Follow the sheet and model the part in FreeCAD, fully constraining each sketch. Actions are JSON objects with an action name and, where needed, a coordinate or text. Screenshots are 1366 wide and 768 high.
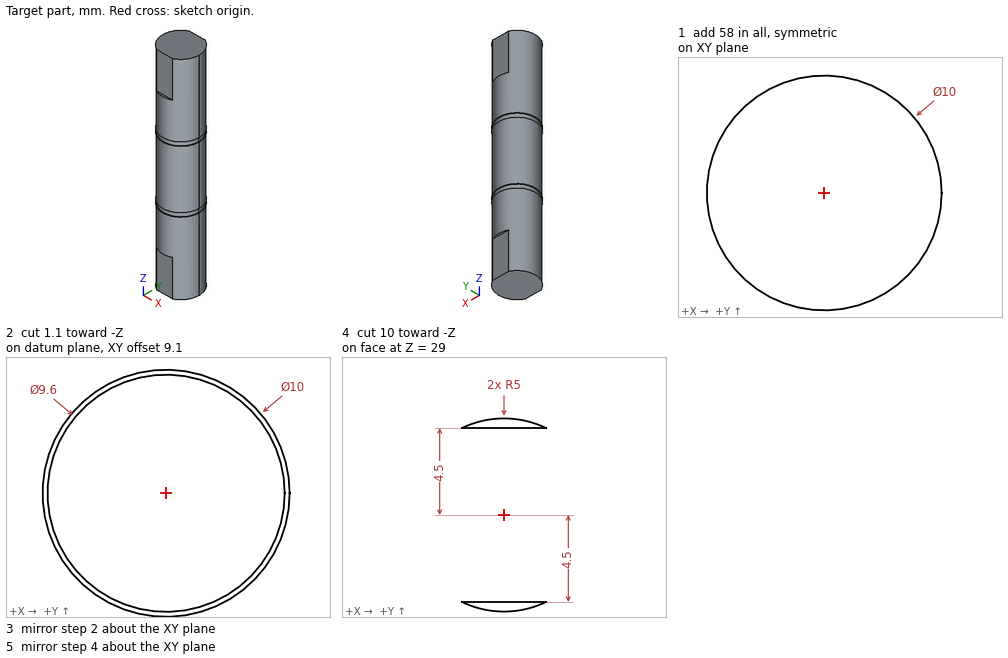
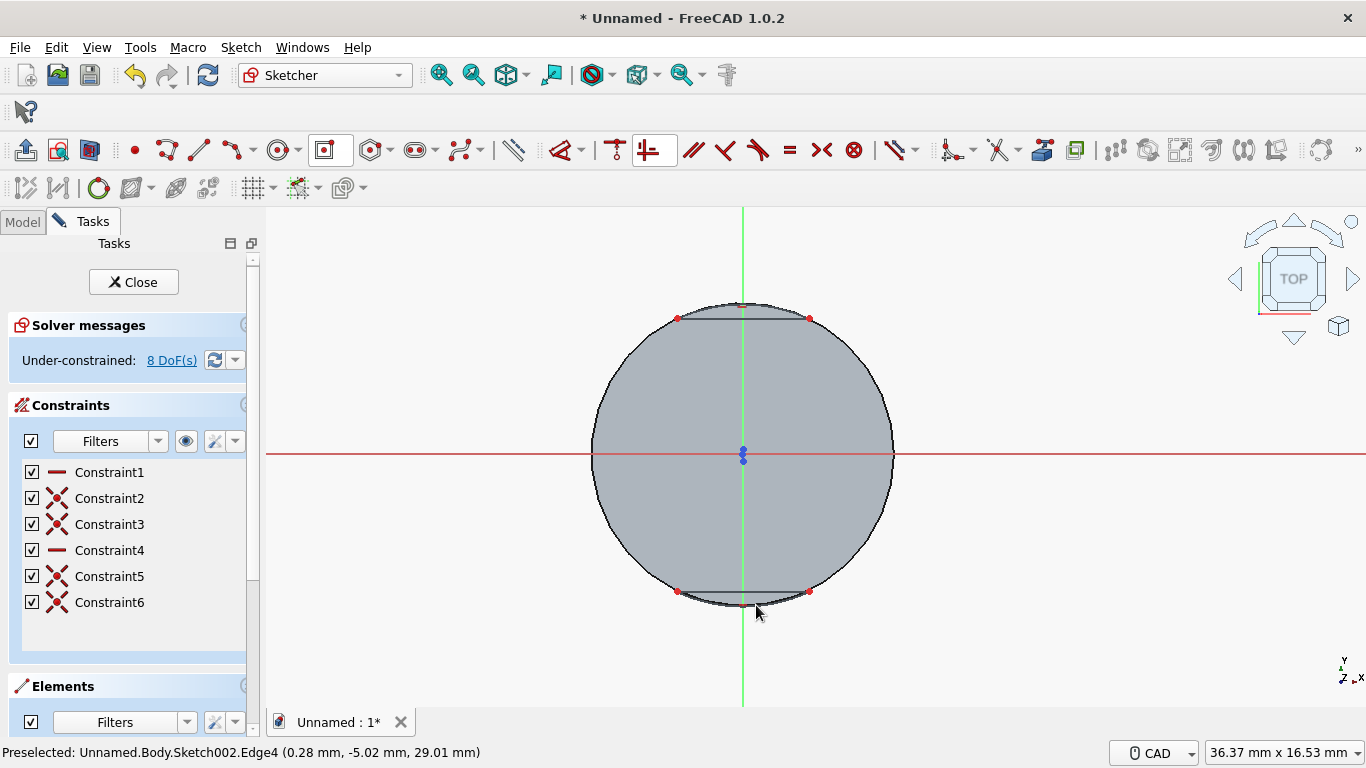
{"action": "left_click", "coordinate": [770, 307]}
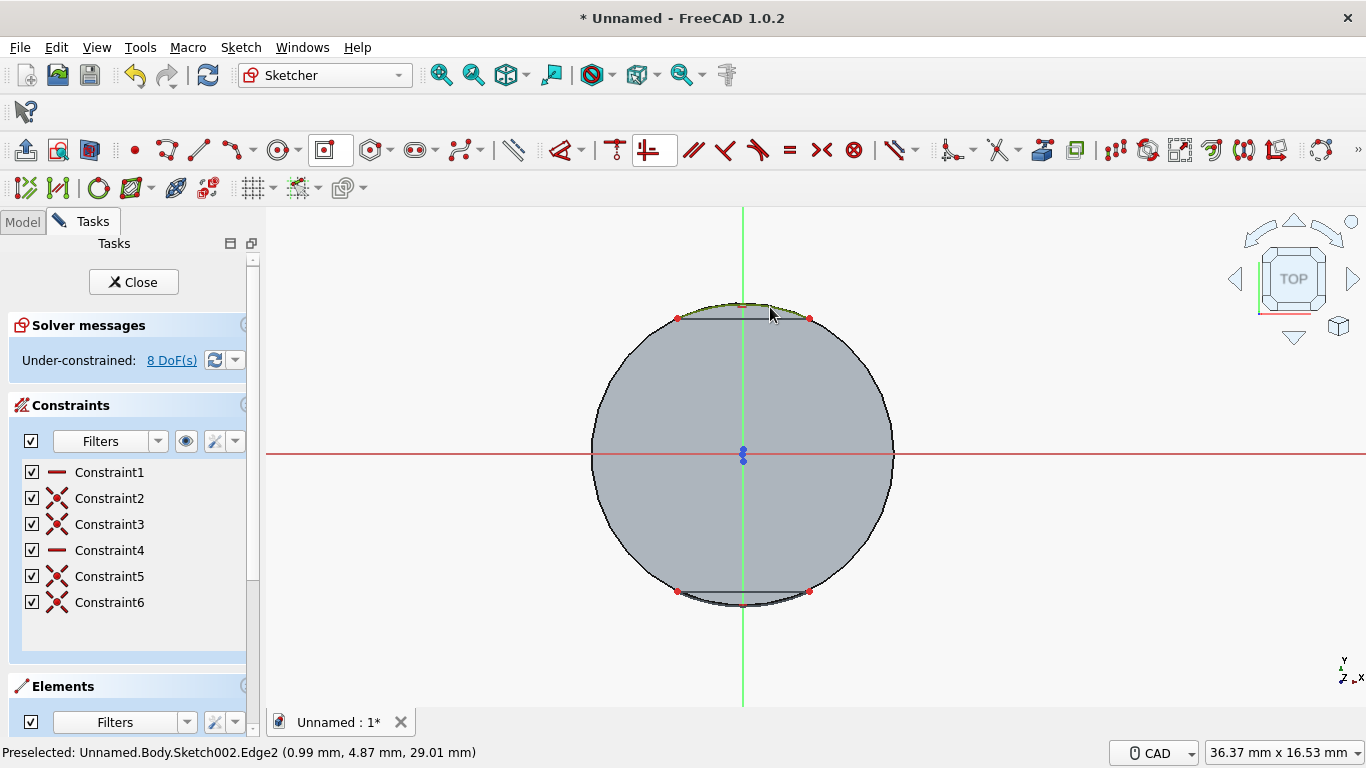
{"action": "left_click", "coordinate": [716, 604]}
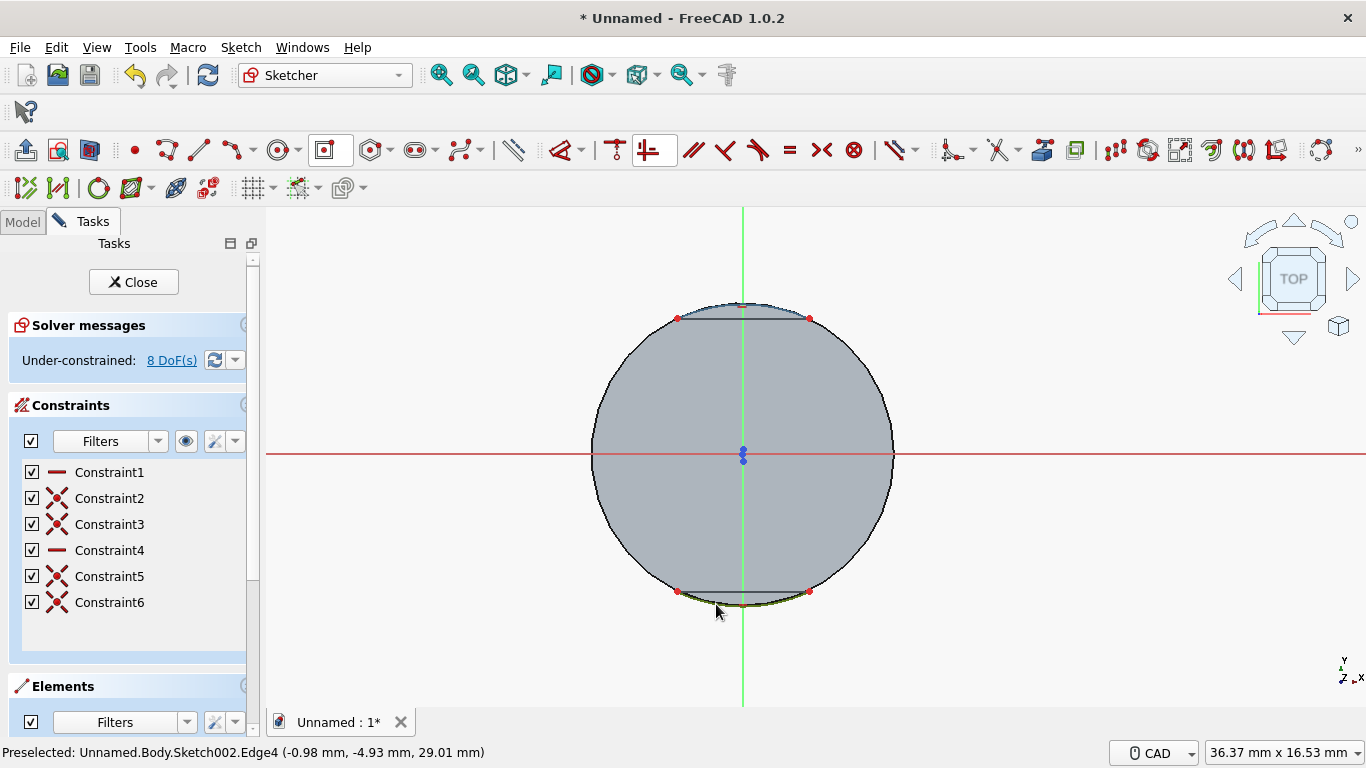
{"action": "left_click", "coordinate": [616, 150]}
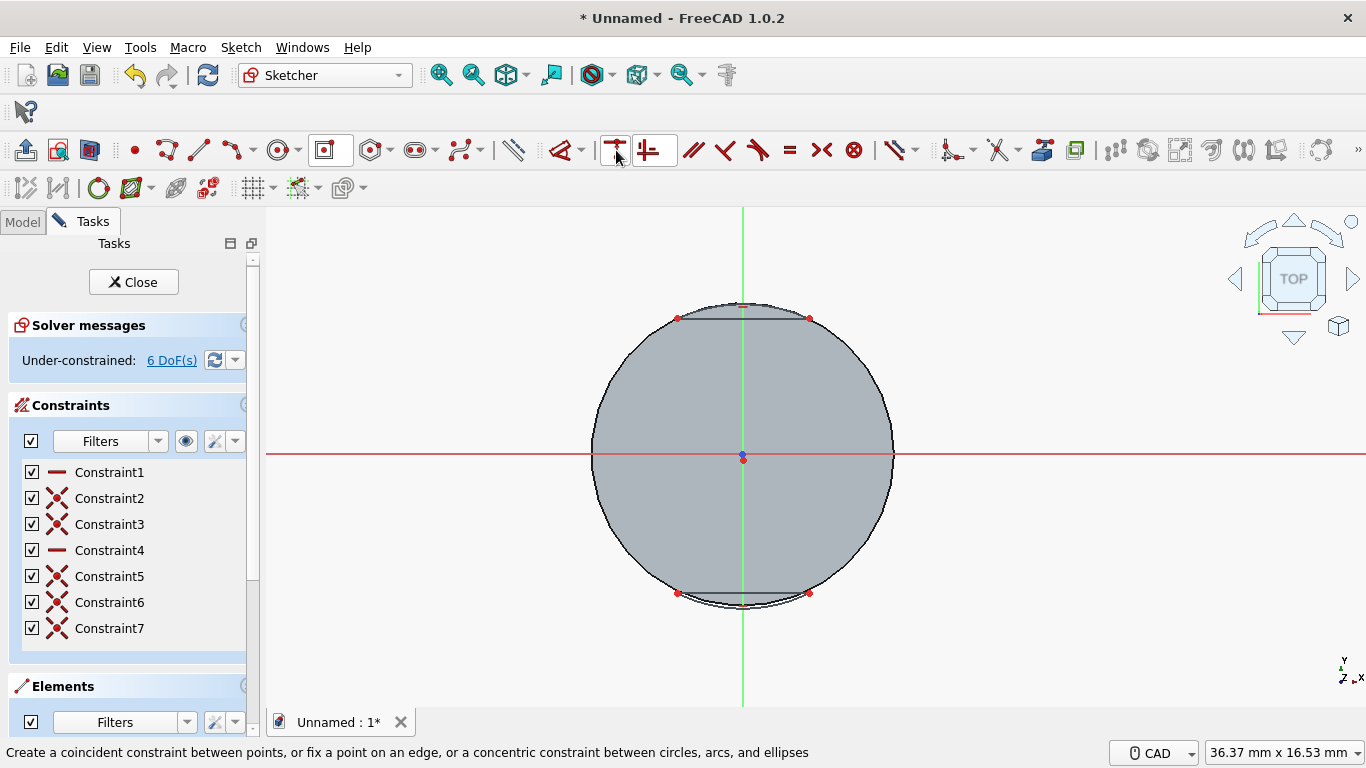
{"action": "left_click_drag", "start_coordinate": [733, 444], "coordinate": [753, 470]}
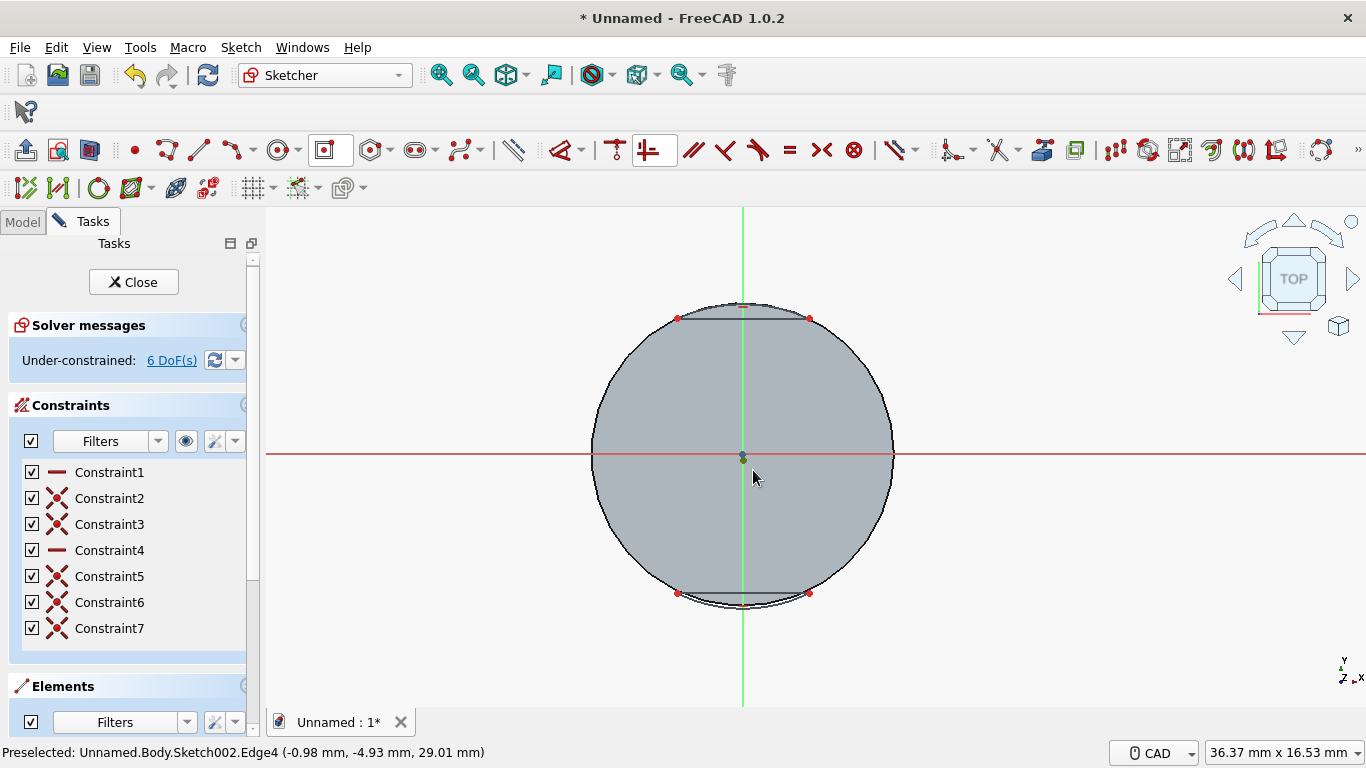
{"action": "left_click", "coordinate": [616, 150]}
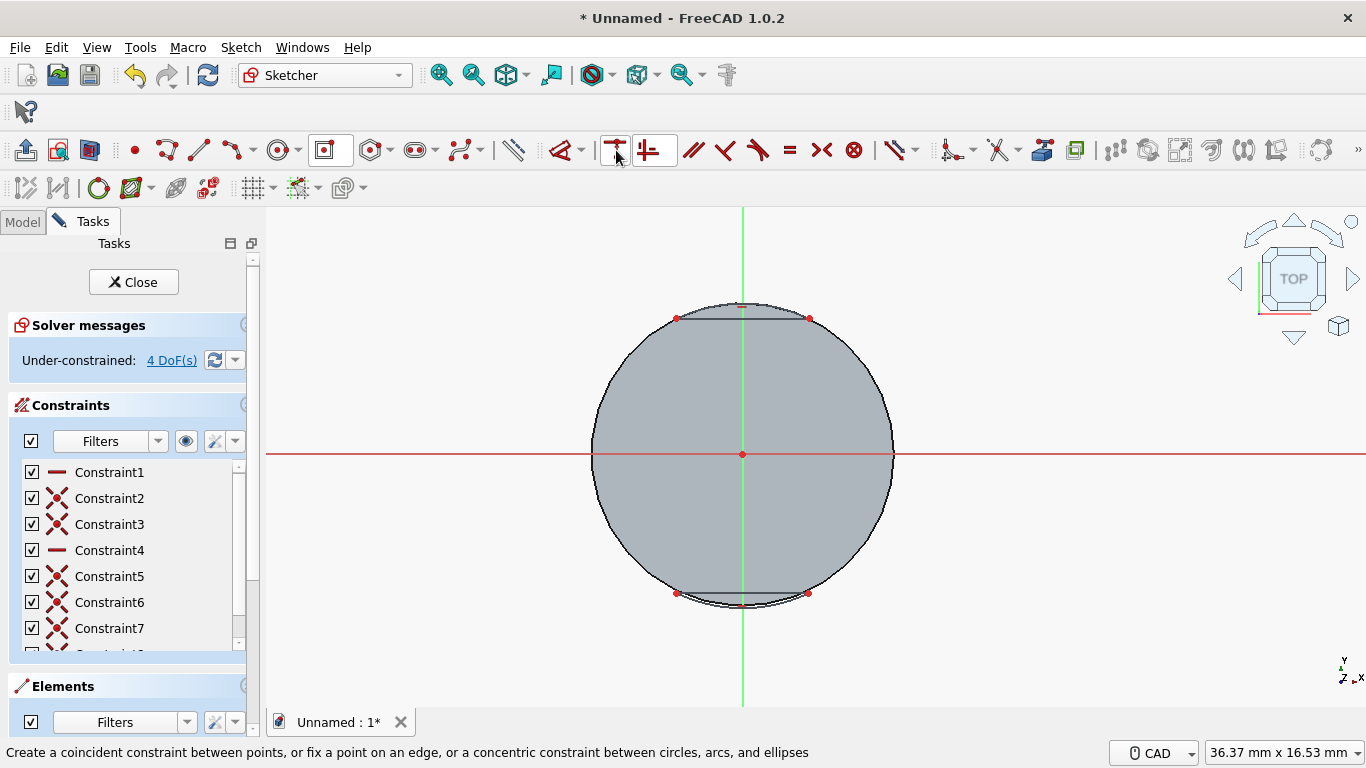
{"action": "left_click", "coordinate": [770, 306]}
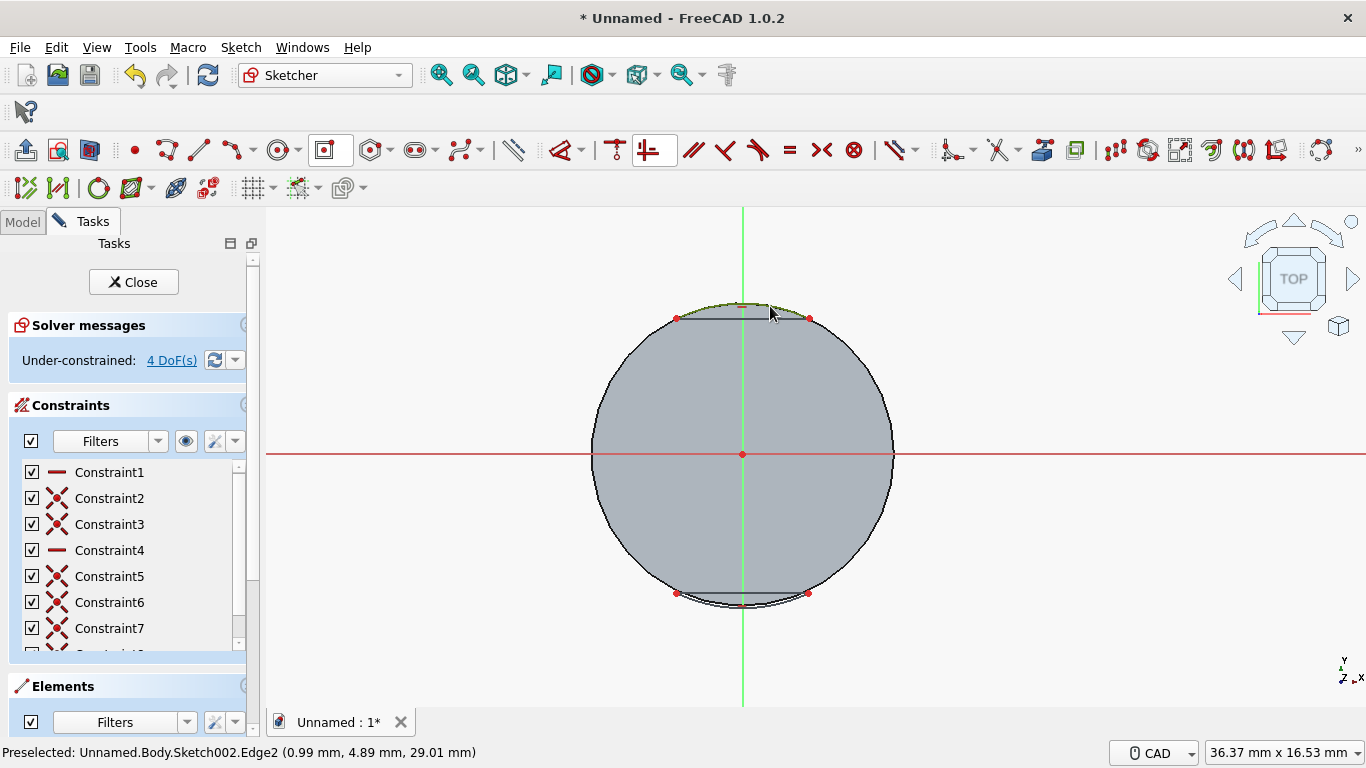
{"action": "left_click", "coordinate": [716, 606]}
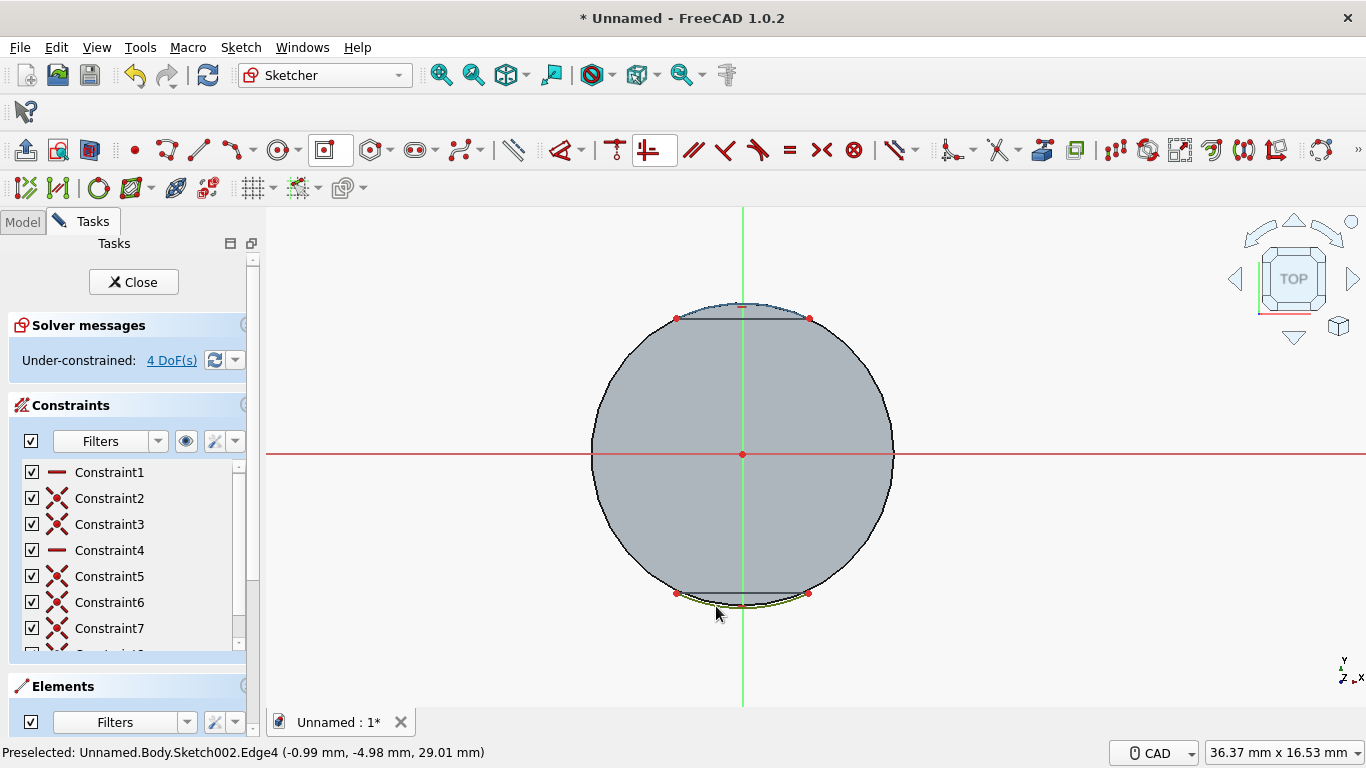
{"action": "left_click", "coordinate": [790, 150]}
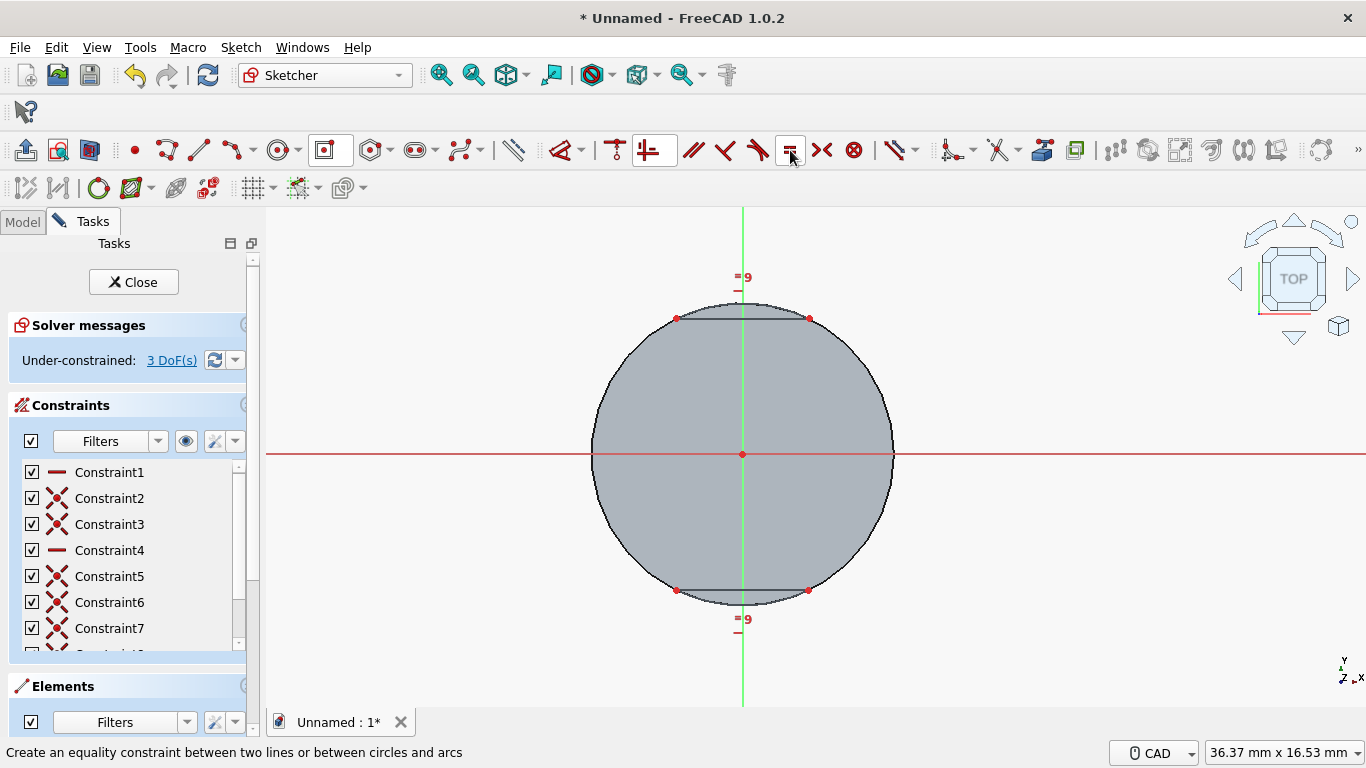
{"action": "left_click", "coordinate": [560, 150]}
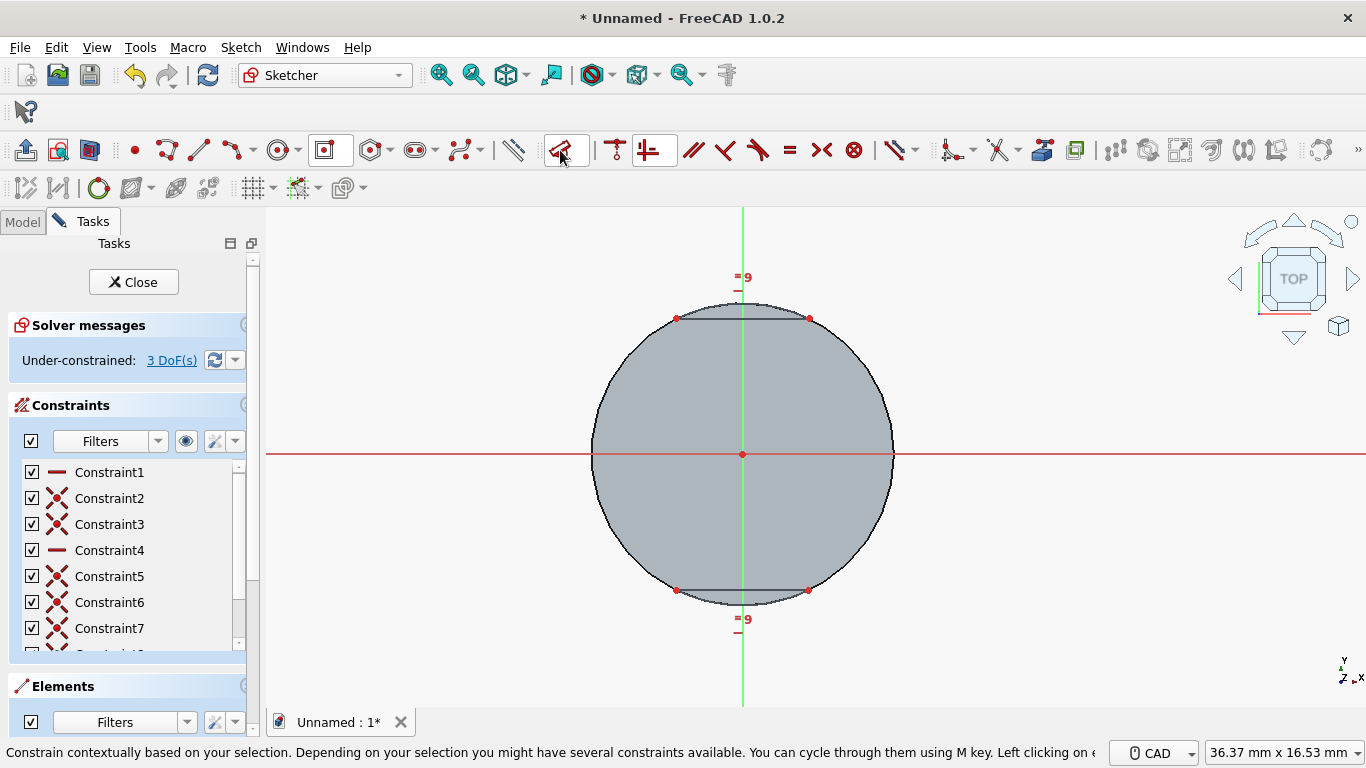
{"action": "left_click", "coordinate": [770, 306]}
{"action": "left_click", "coordinate": [776, 275]}